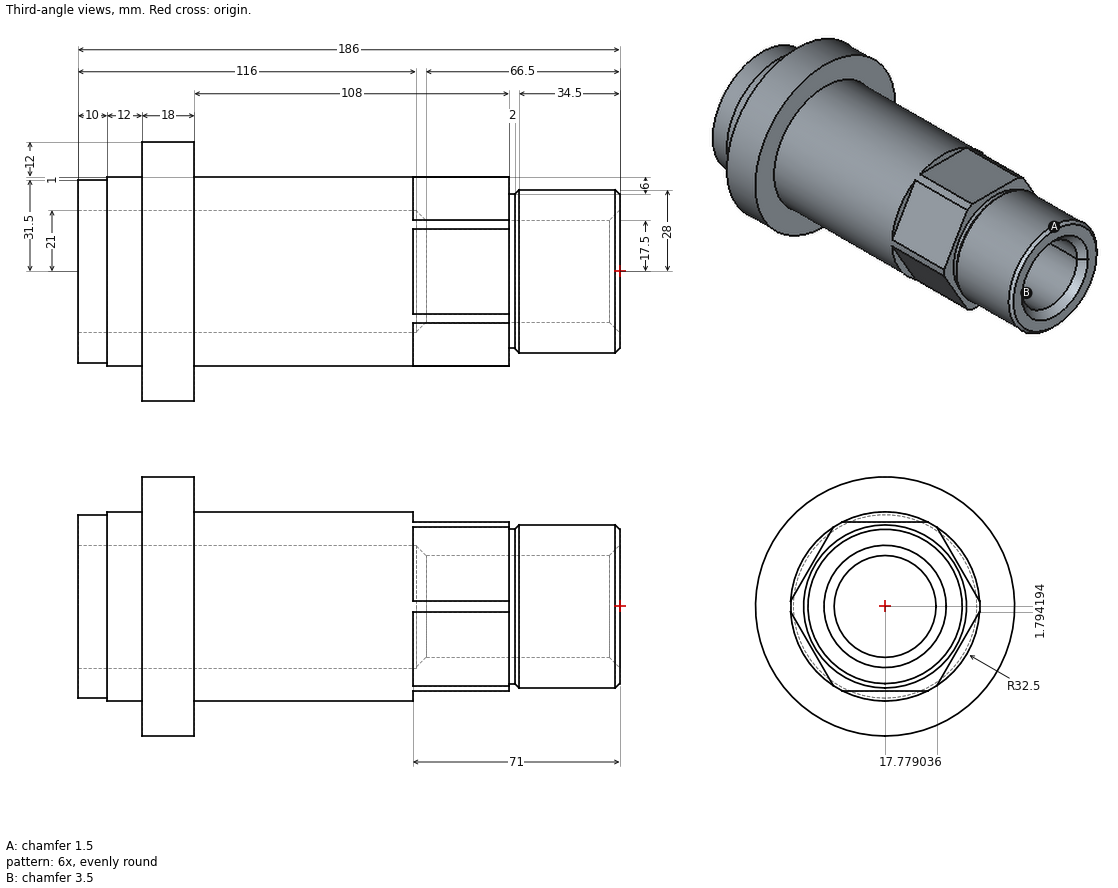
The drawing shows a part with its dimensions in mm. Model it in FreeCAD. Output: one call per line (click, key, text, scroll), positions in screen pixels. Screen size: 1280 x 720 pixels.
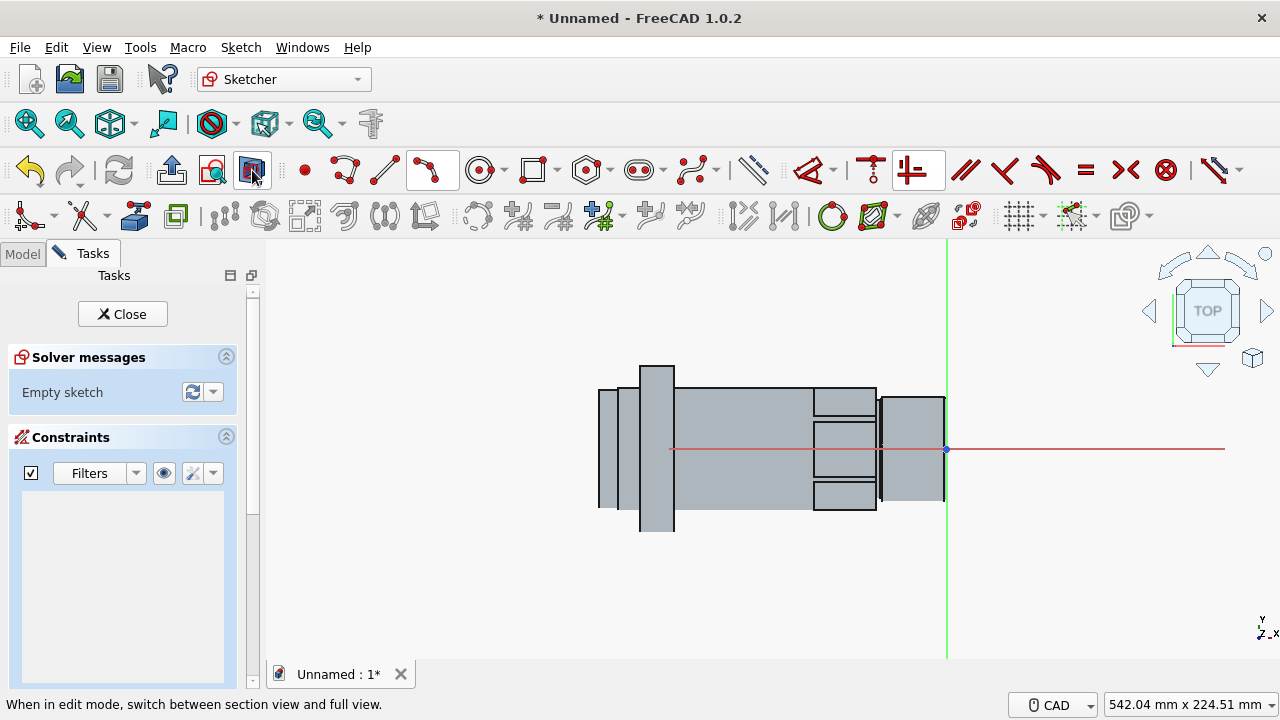
scroll(856, 406, up, 3)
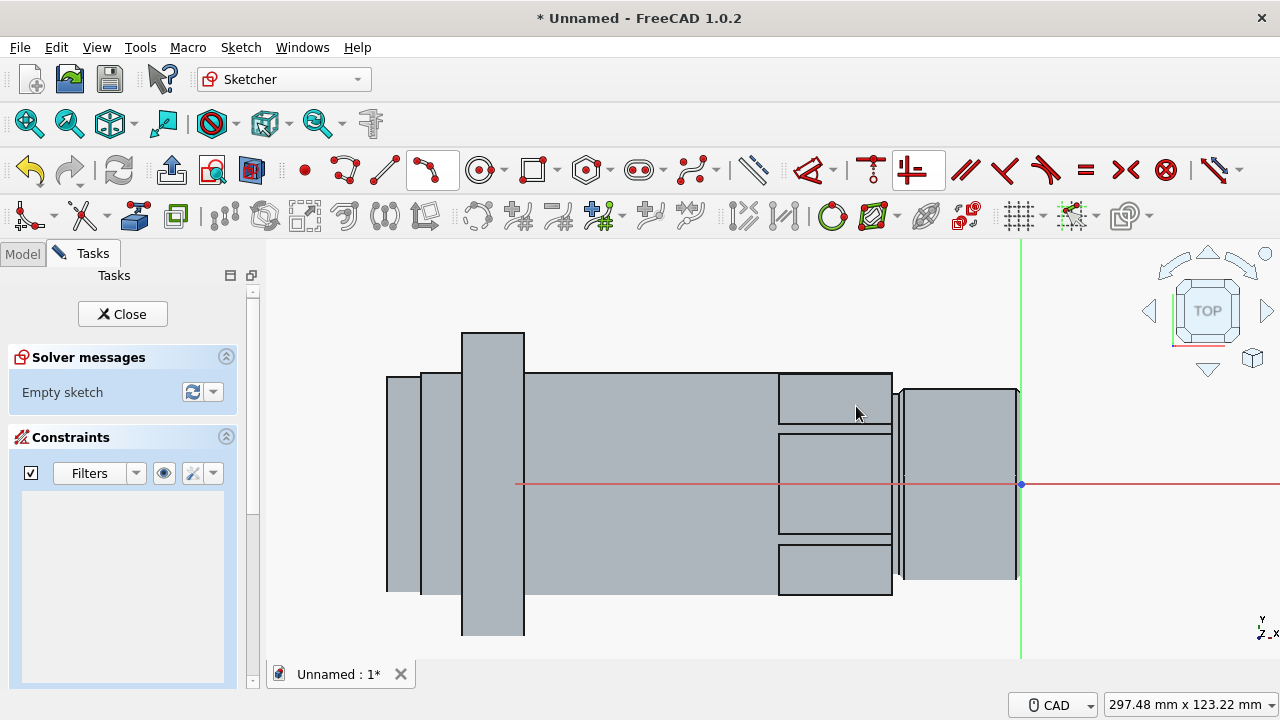
click(346, 170)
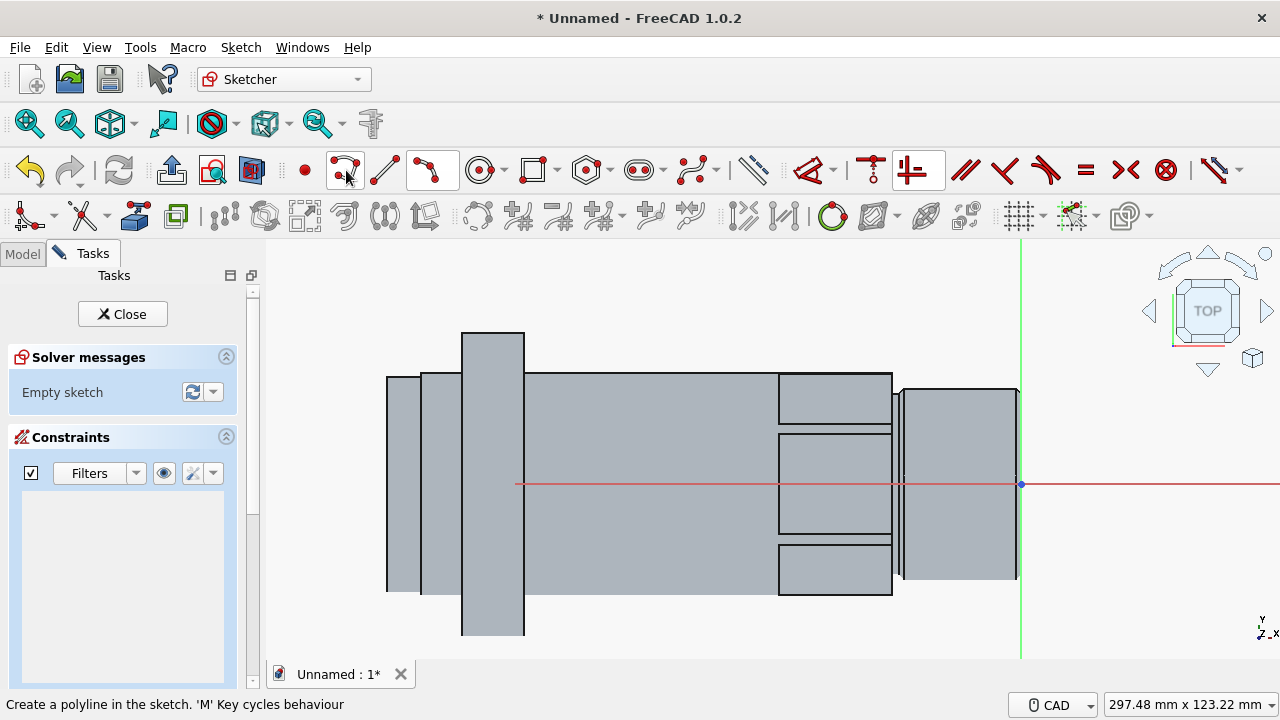
click(1021, 484)
click(1012, 425)
click(795, 425)
click(783, 413)
click(387, 413)
click(387, 475)
click(1021, 484)
key(Escape)
key(Escape)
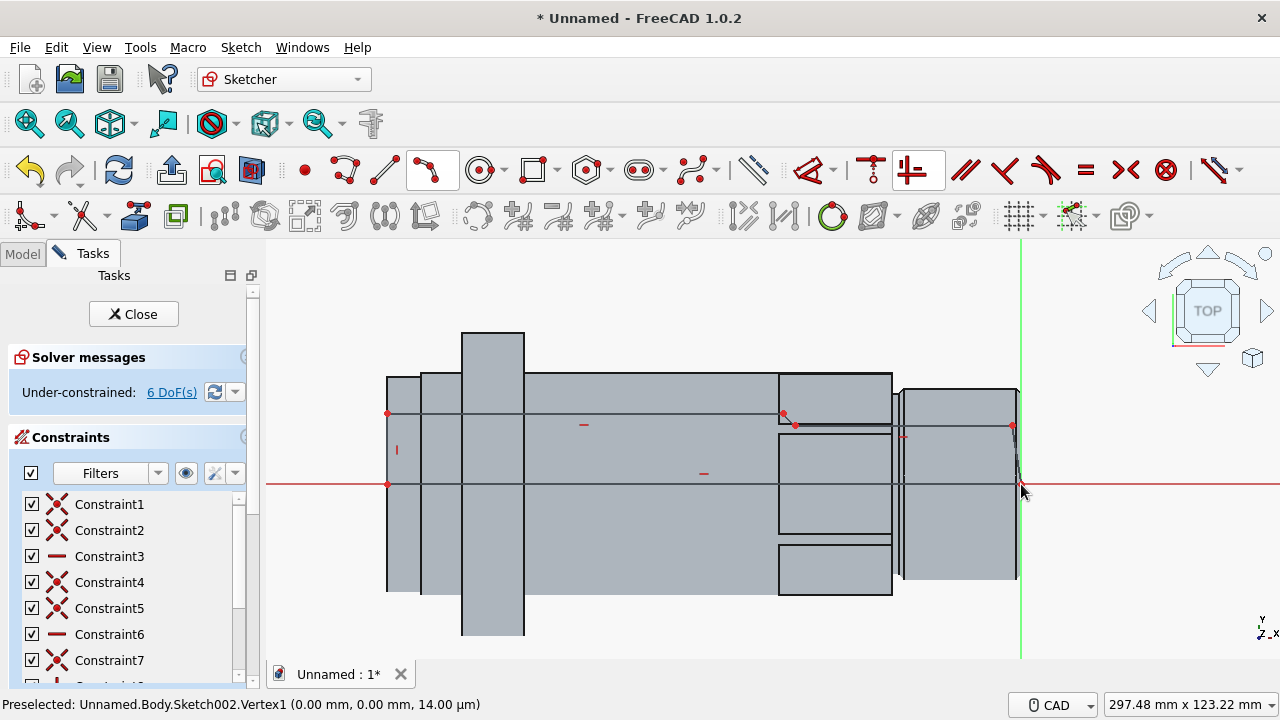
click(1019, 467)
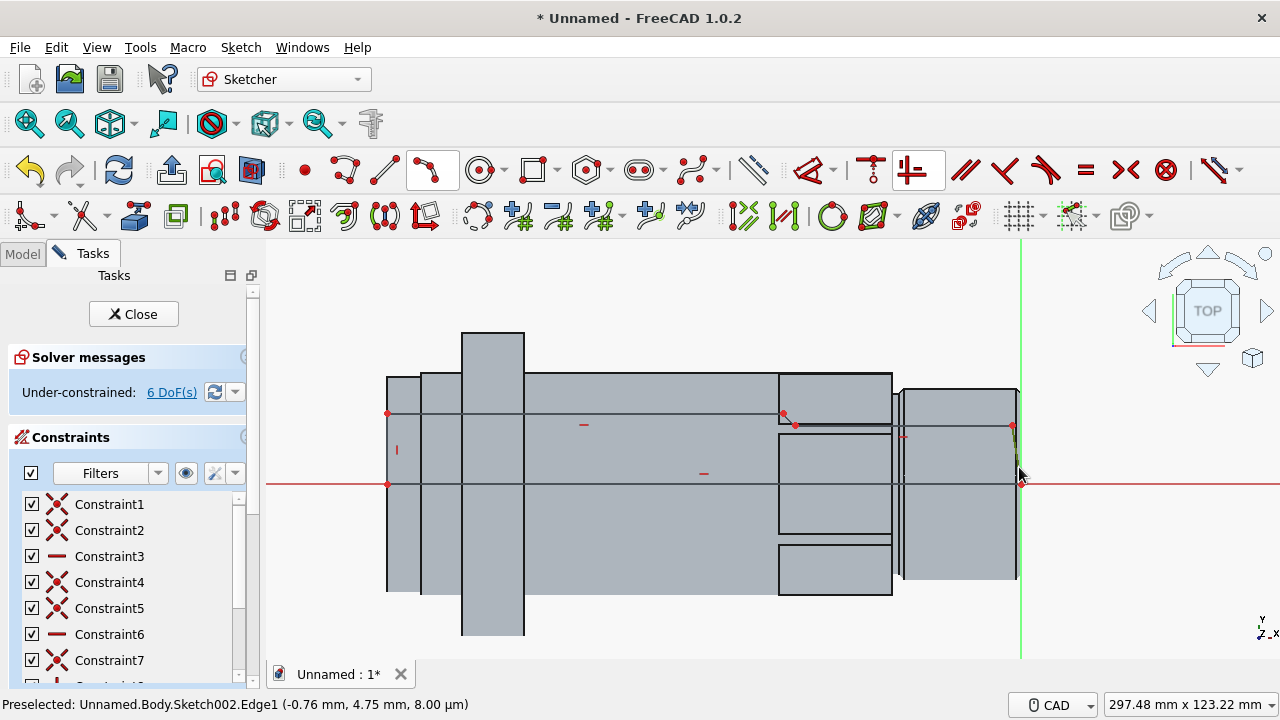
key(v)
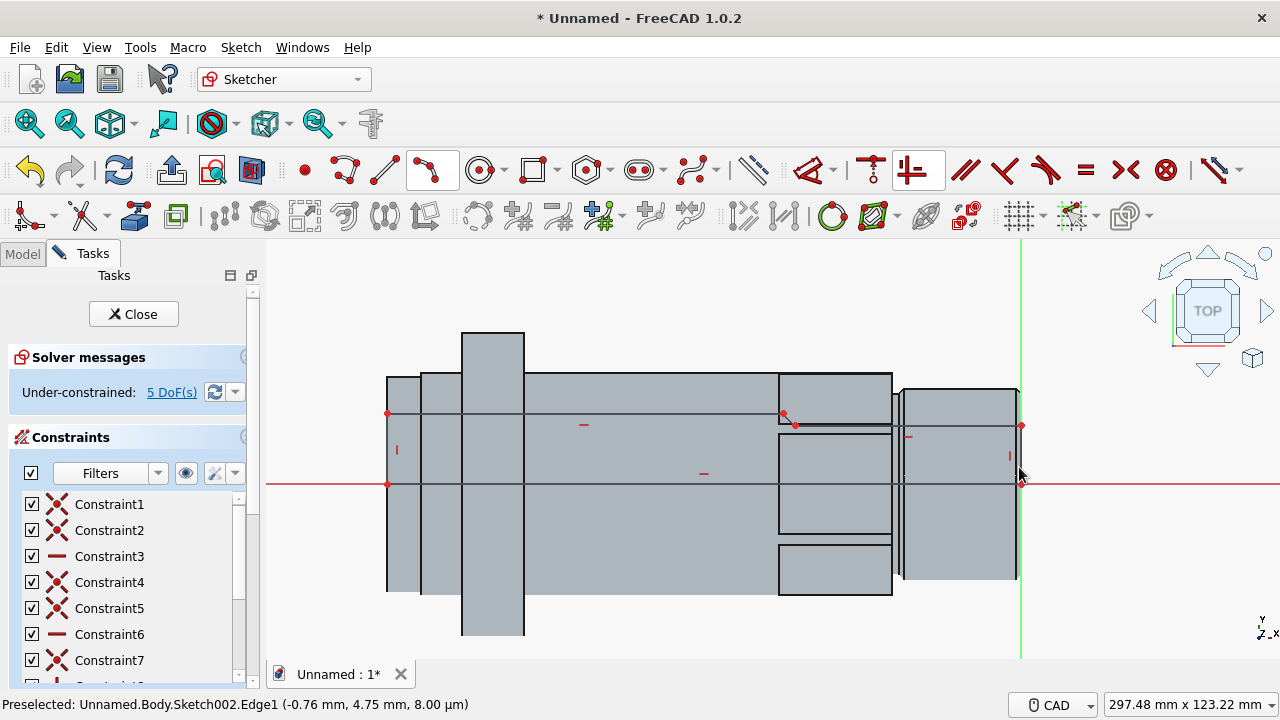
click(808, 170)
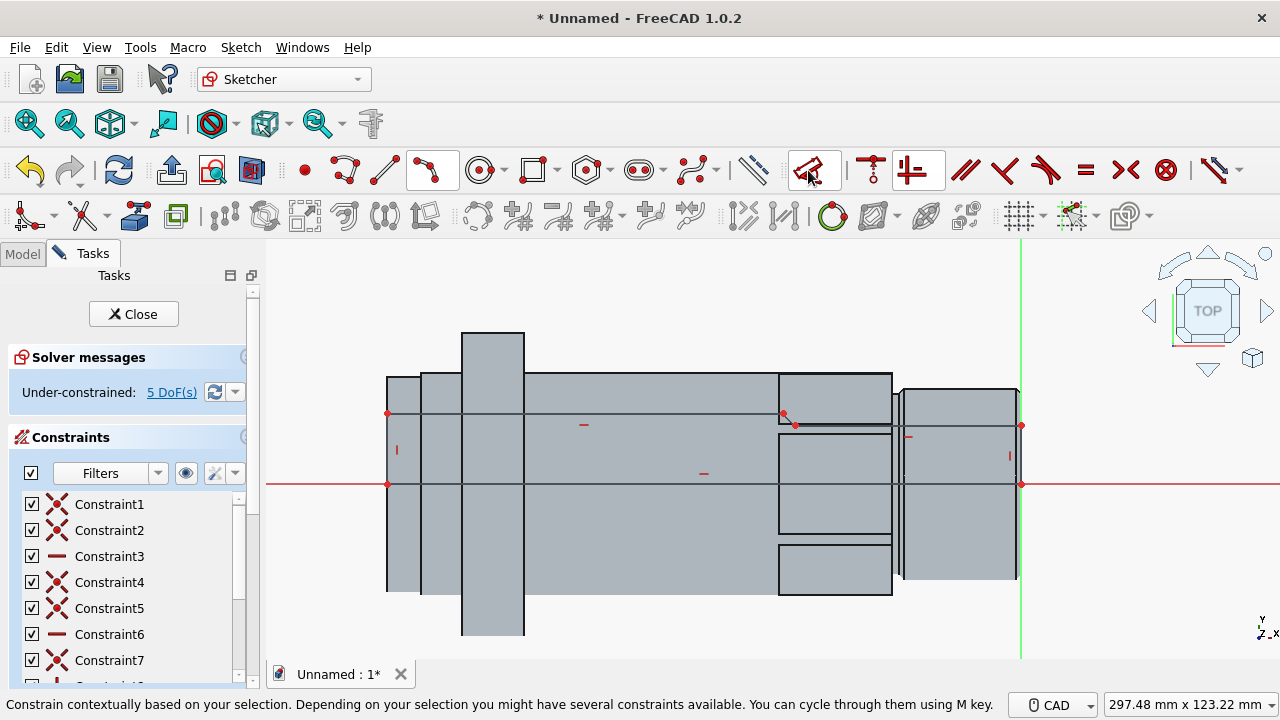
click(387, 435)
click(353, 449)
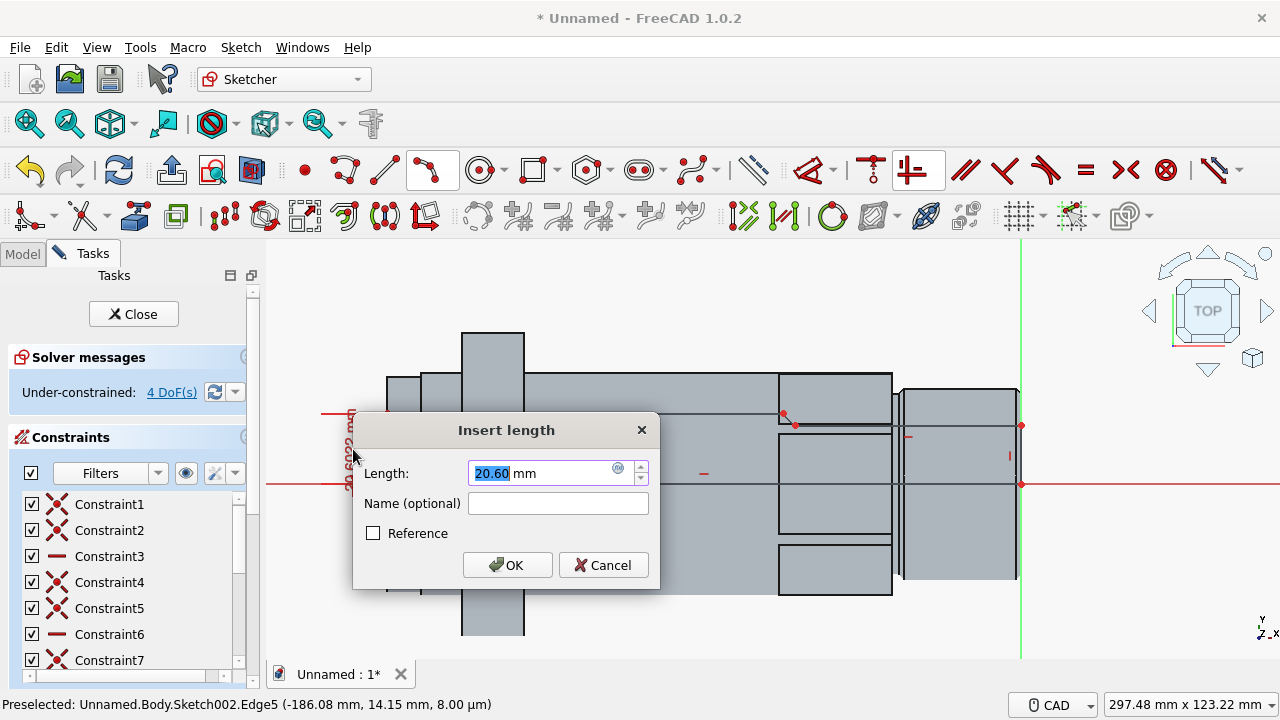
text(21)
key(Return)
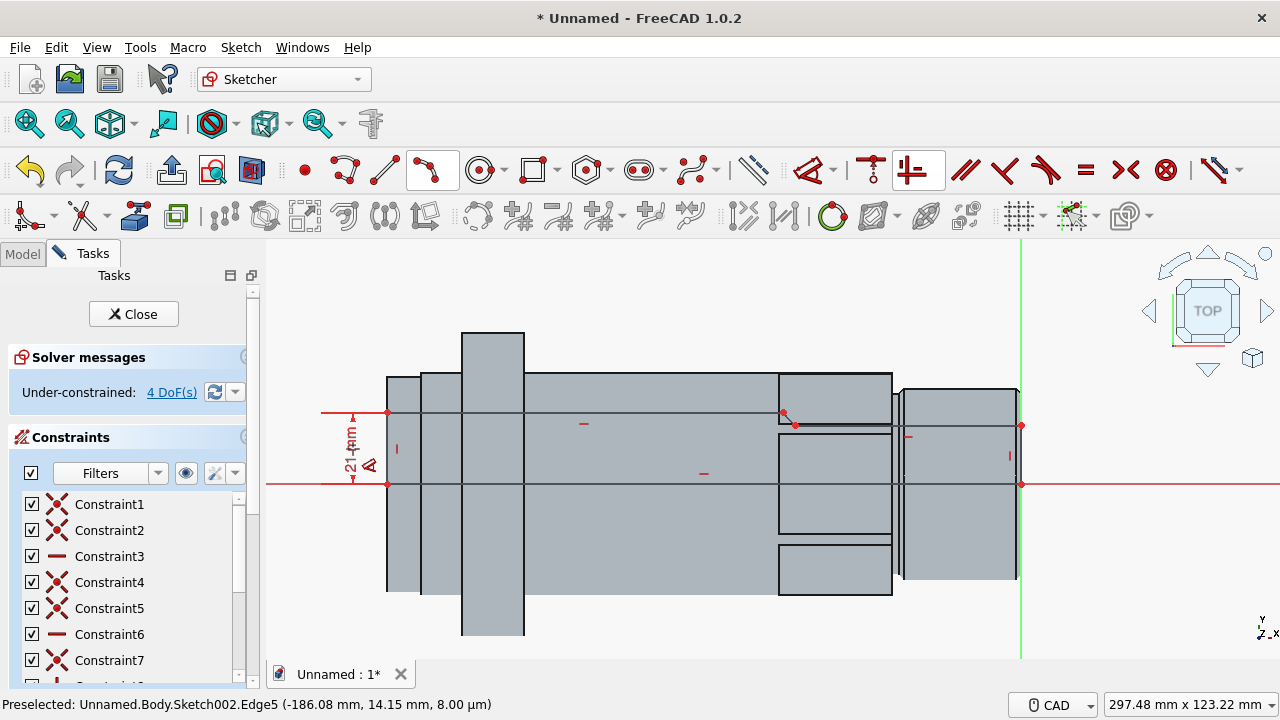
click(664, 413)
click(585, 379)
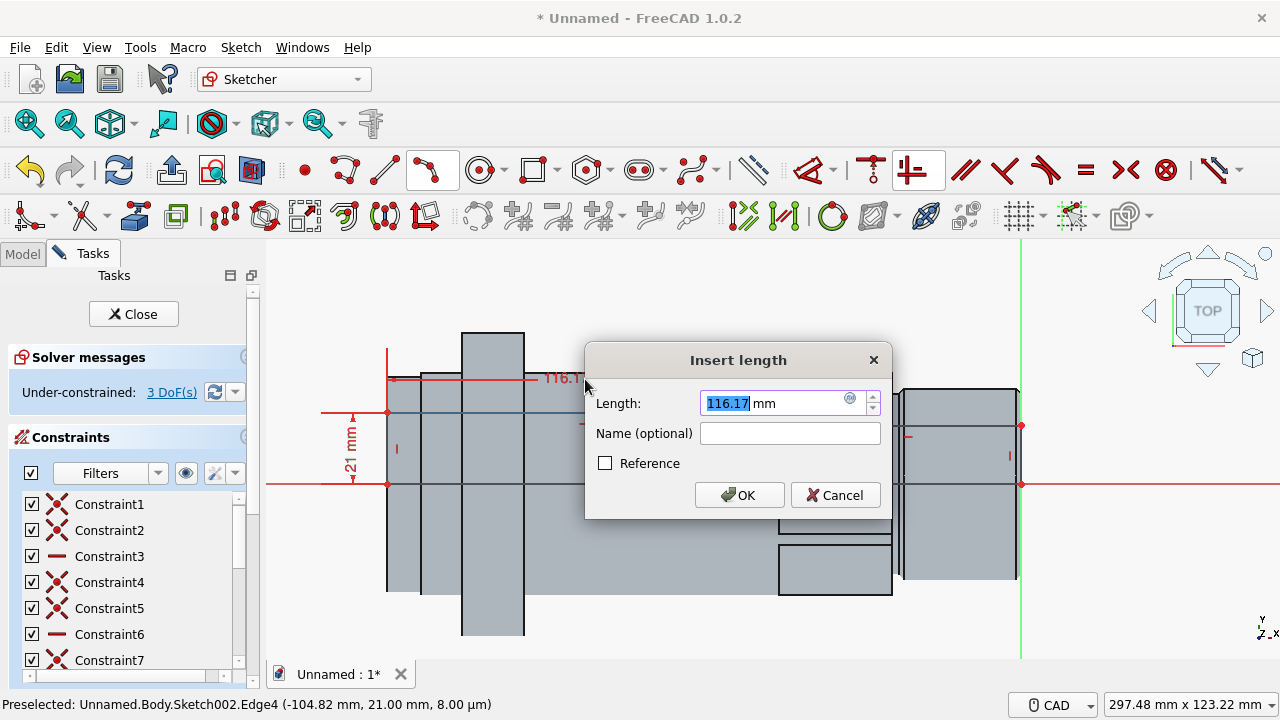
text(116)
key(Return)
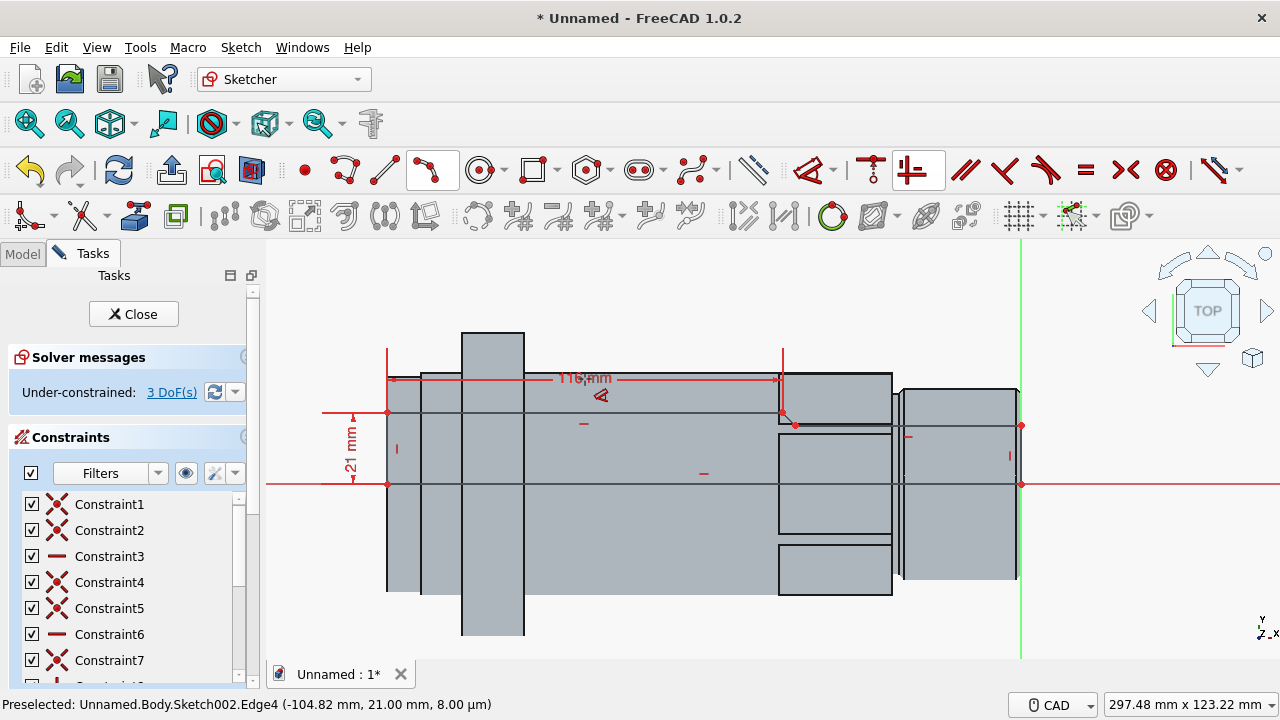
click(577, 484)
click(704, 518)